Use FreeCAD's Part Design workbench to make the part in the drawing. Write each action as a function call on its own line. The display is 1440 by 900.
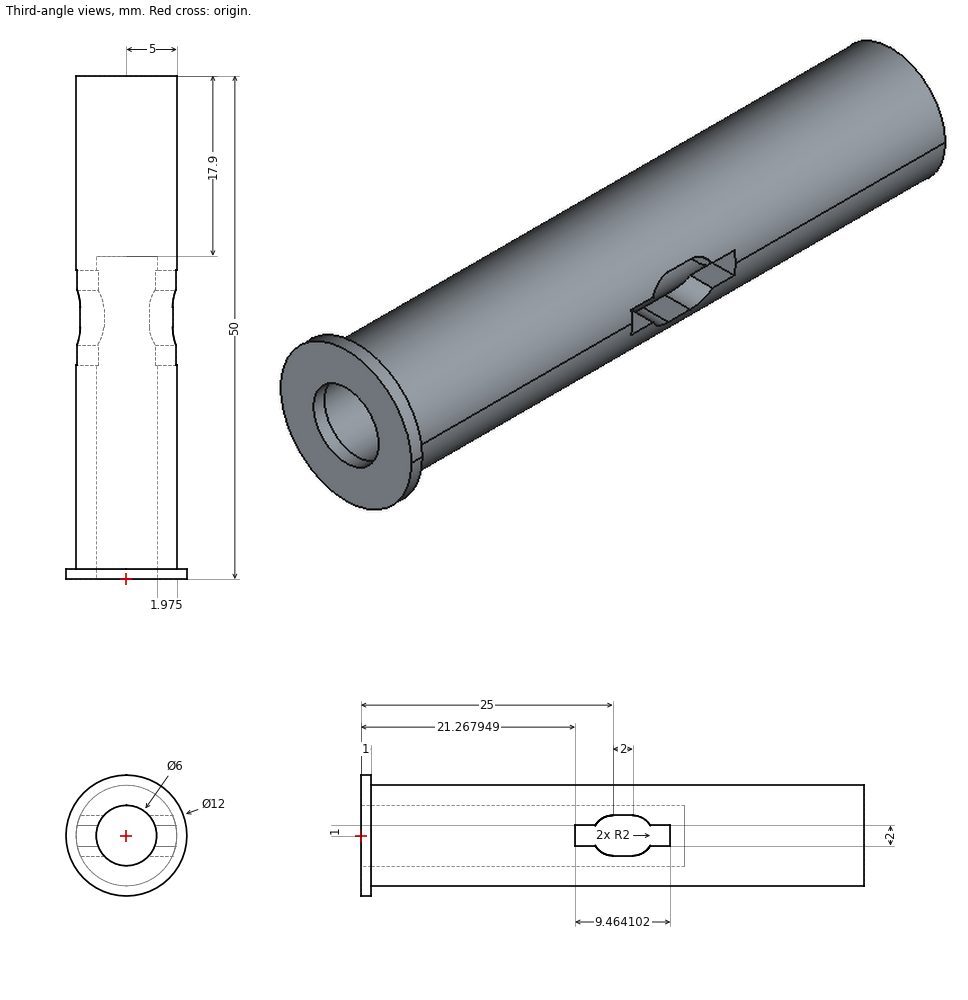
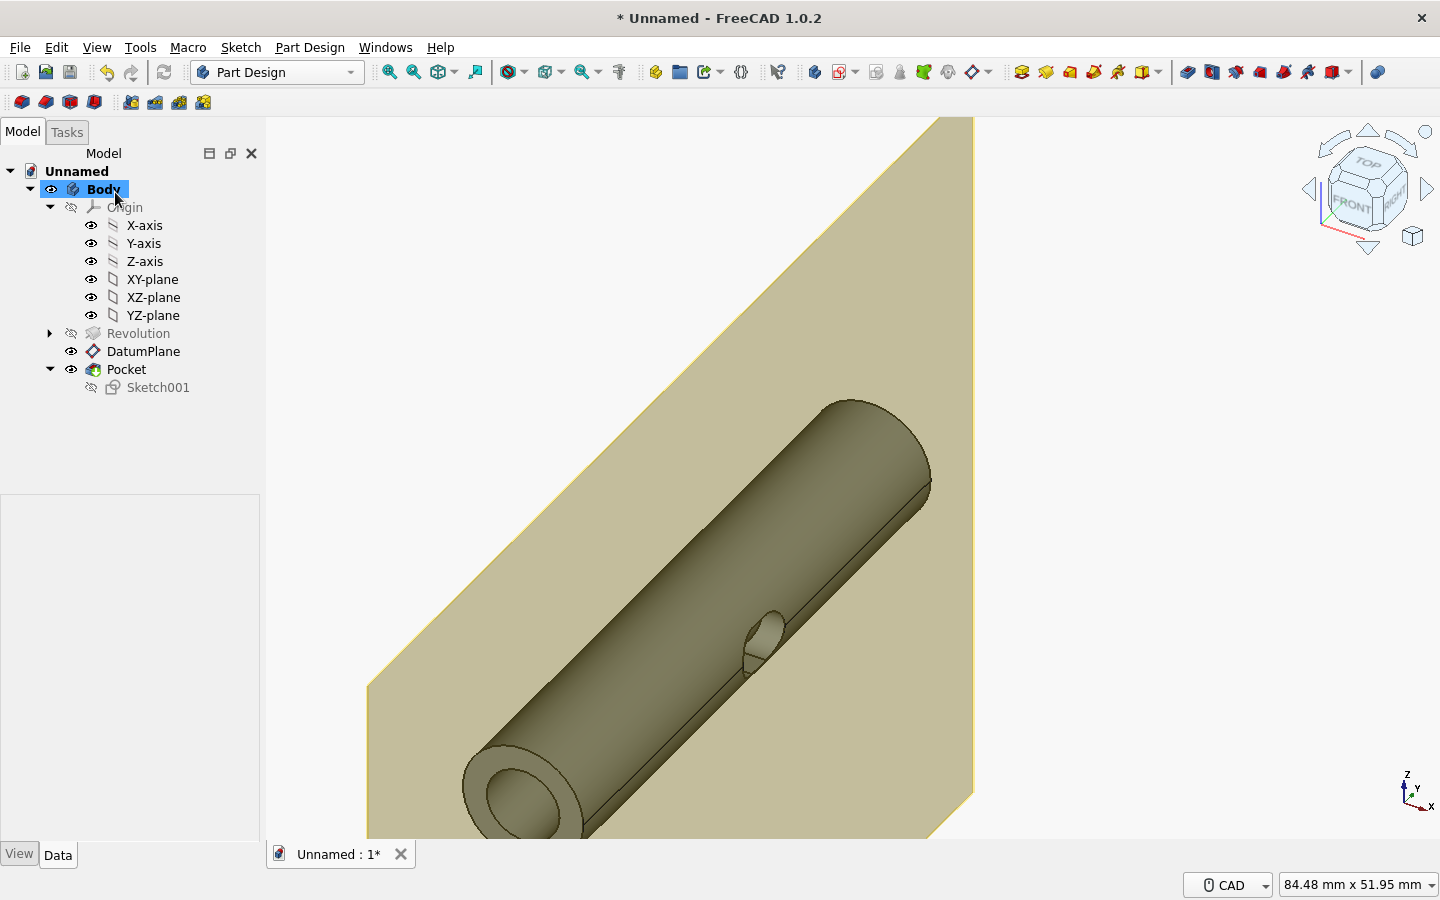
click(116, 351)
key(space)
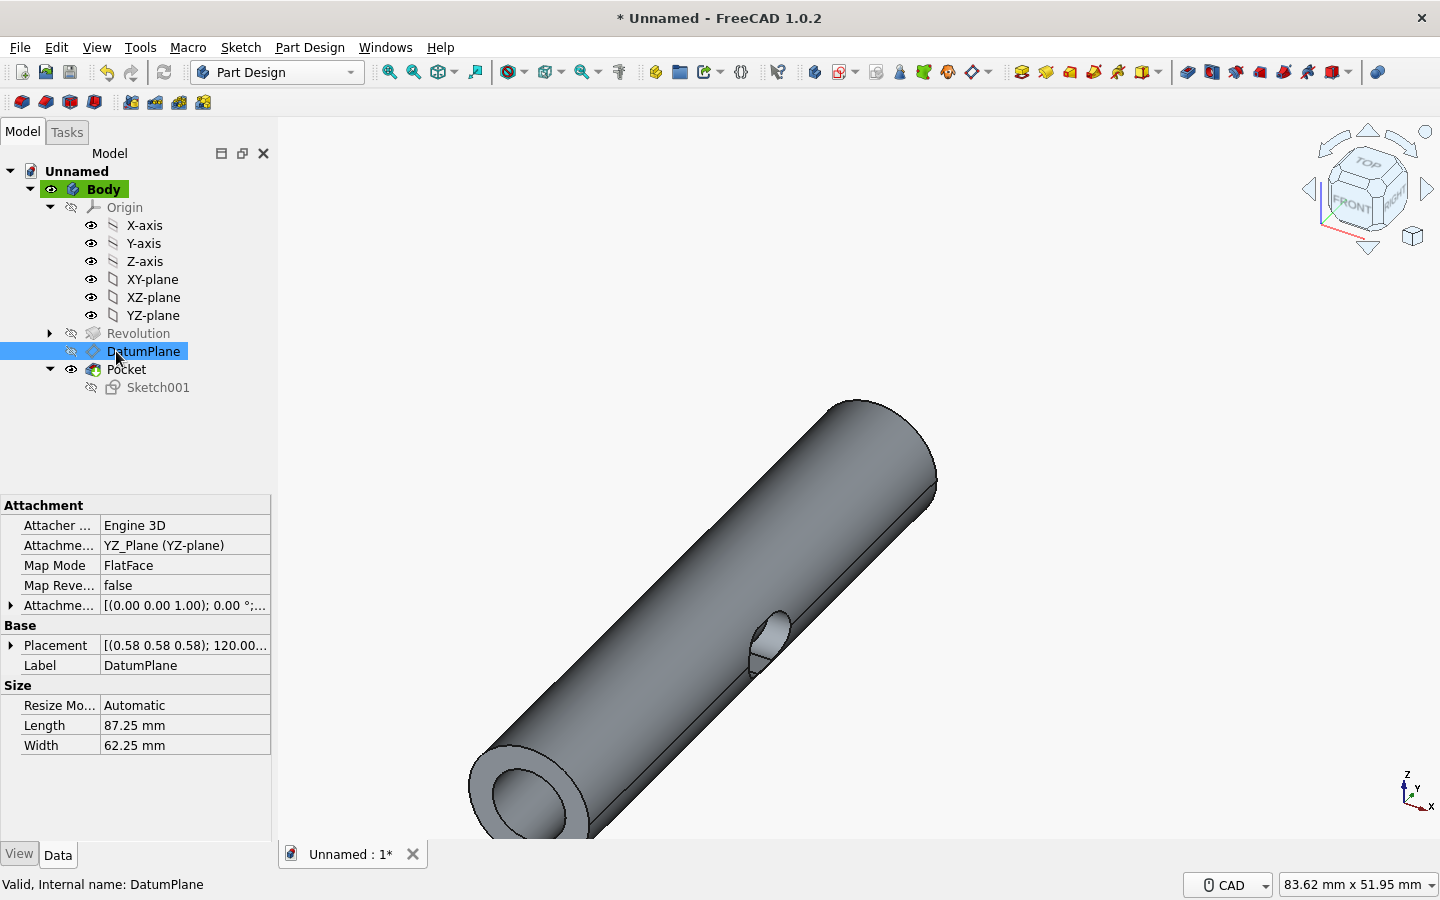
click(390, 72)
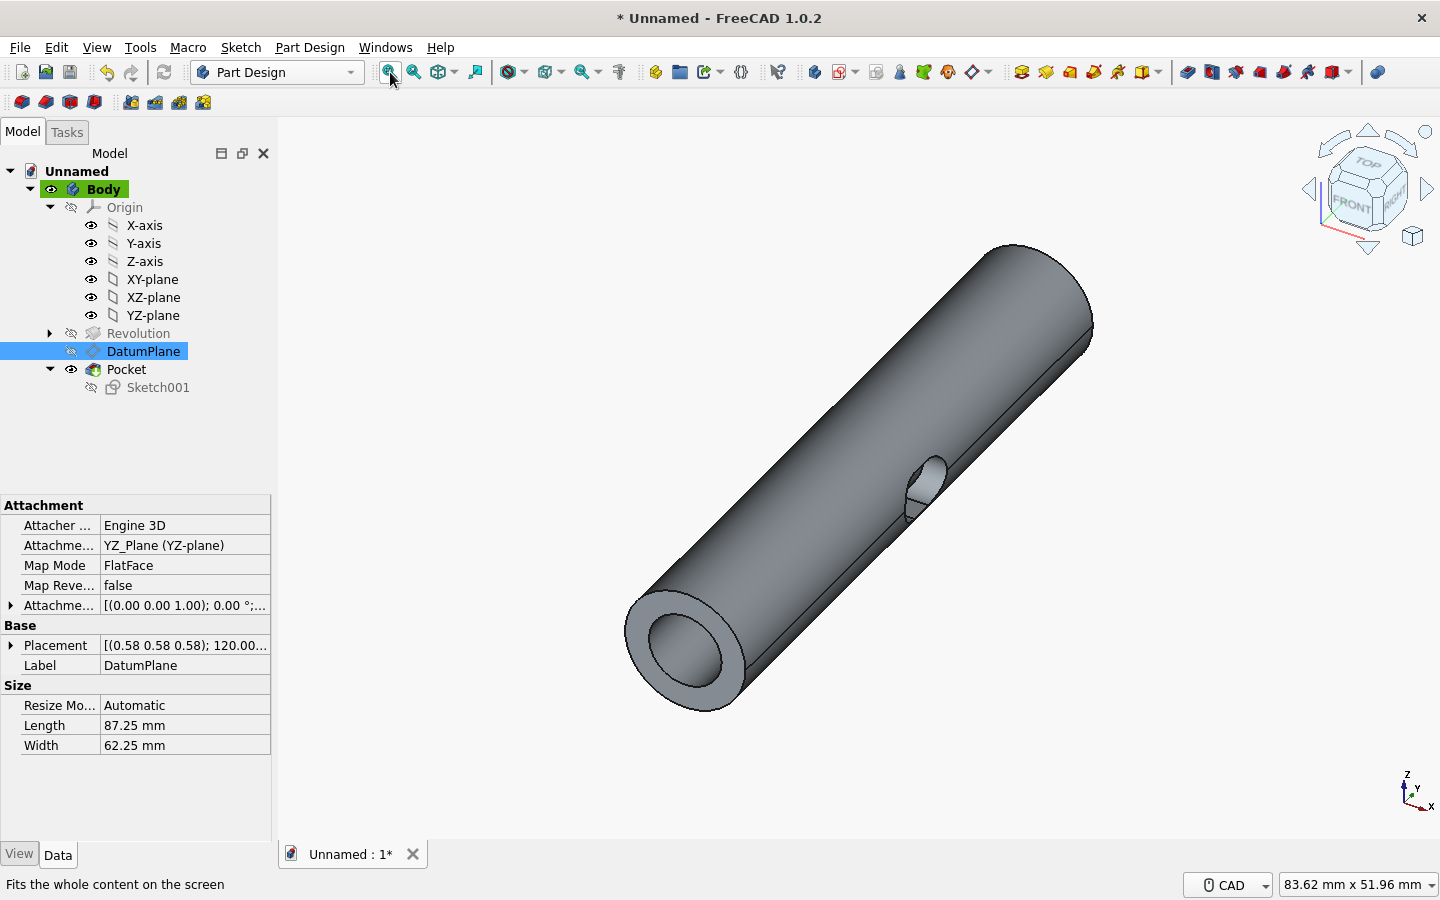
click(318, 799)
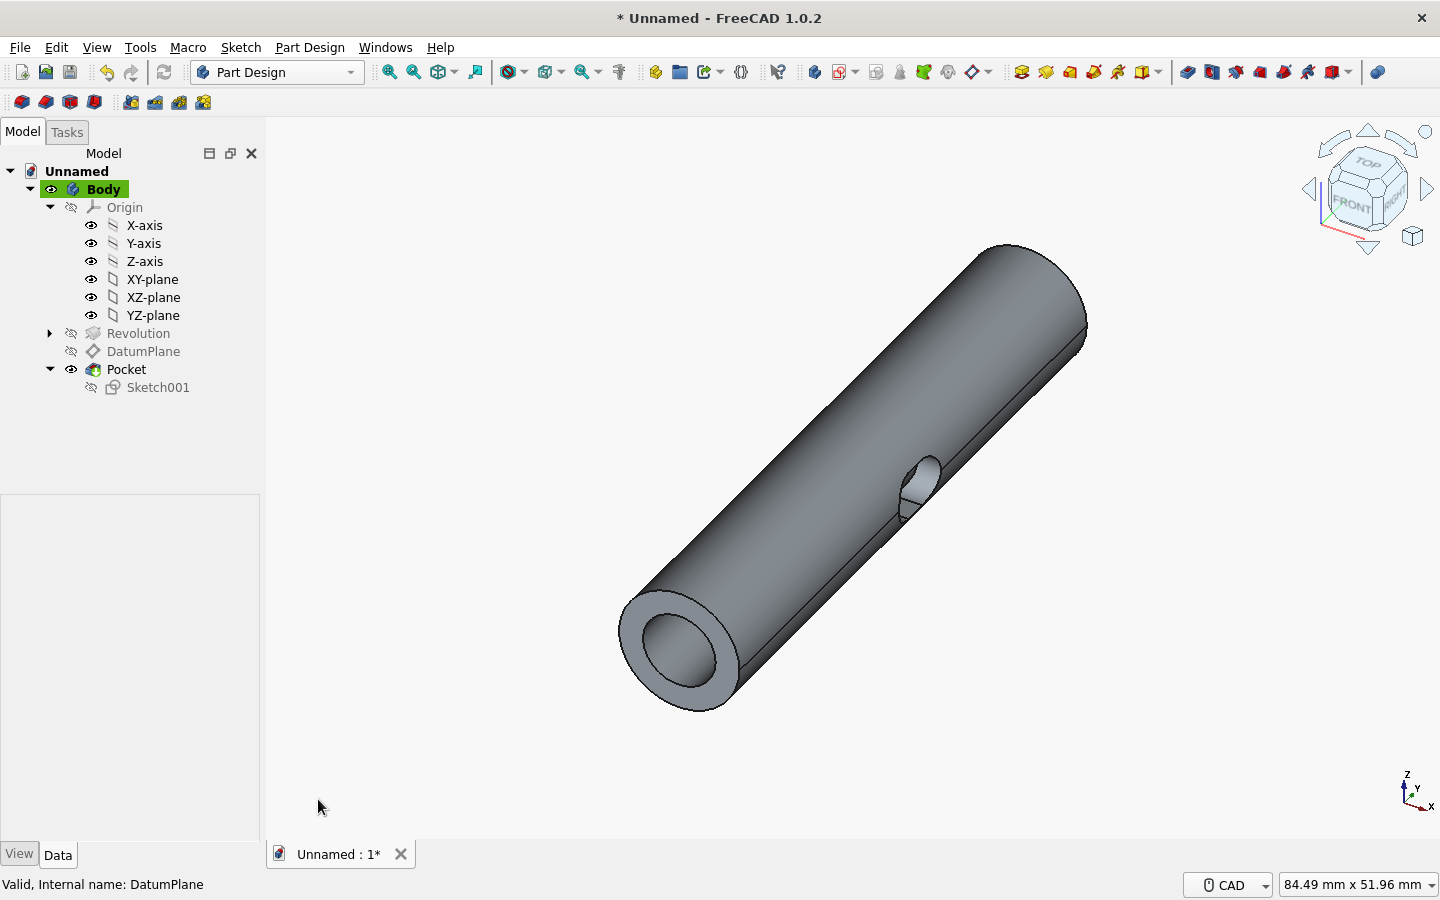
click(840, 72)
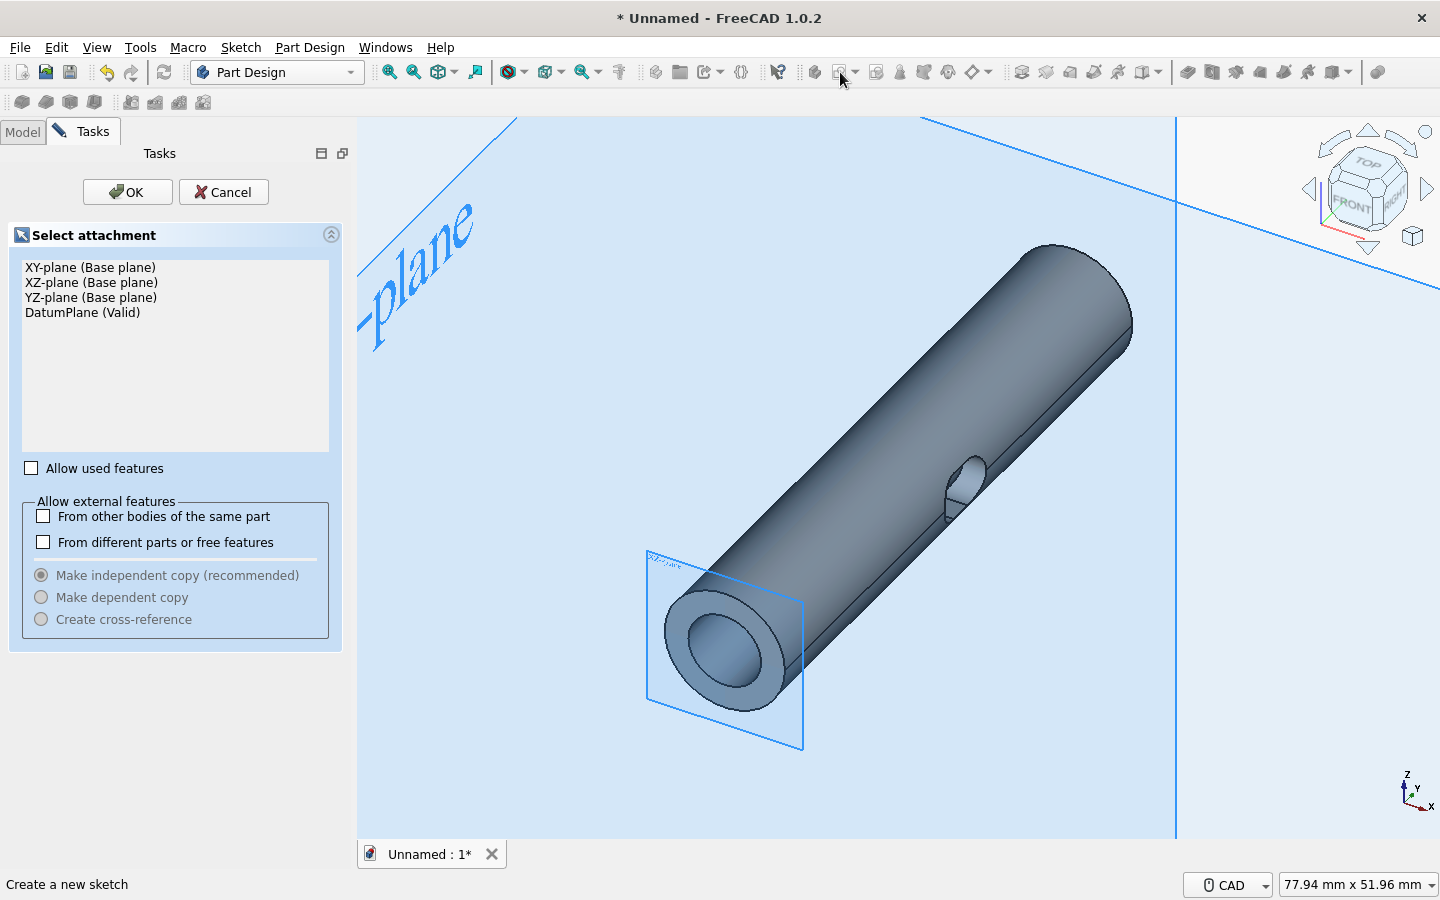
click(82, 282)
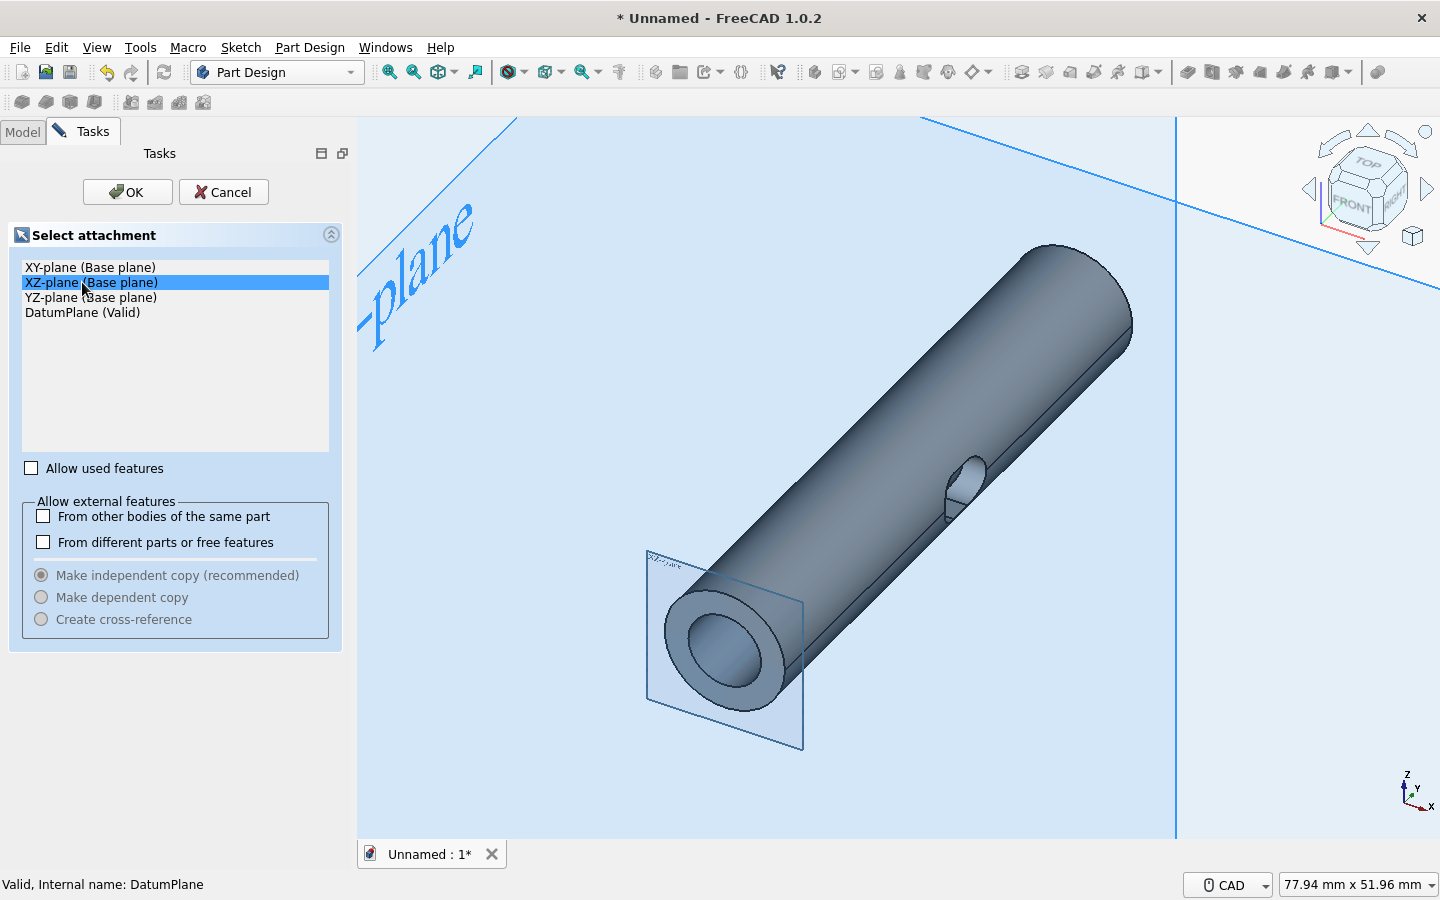
click(128, 192)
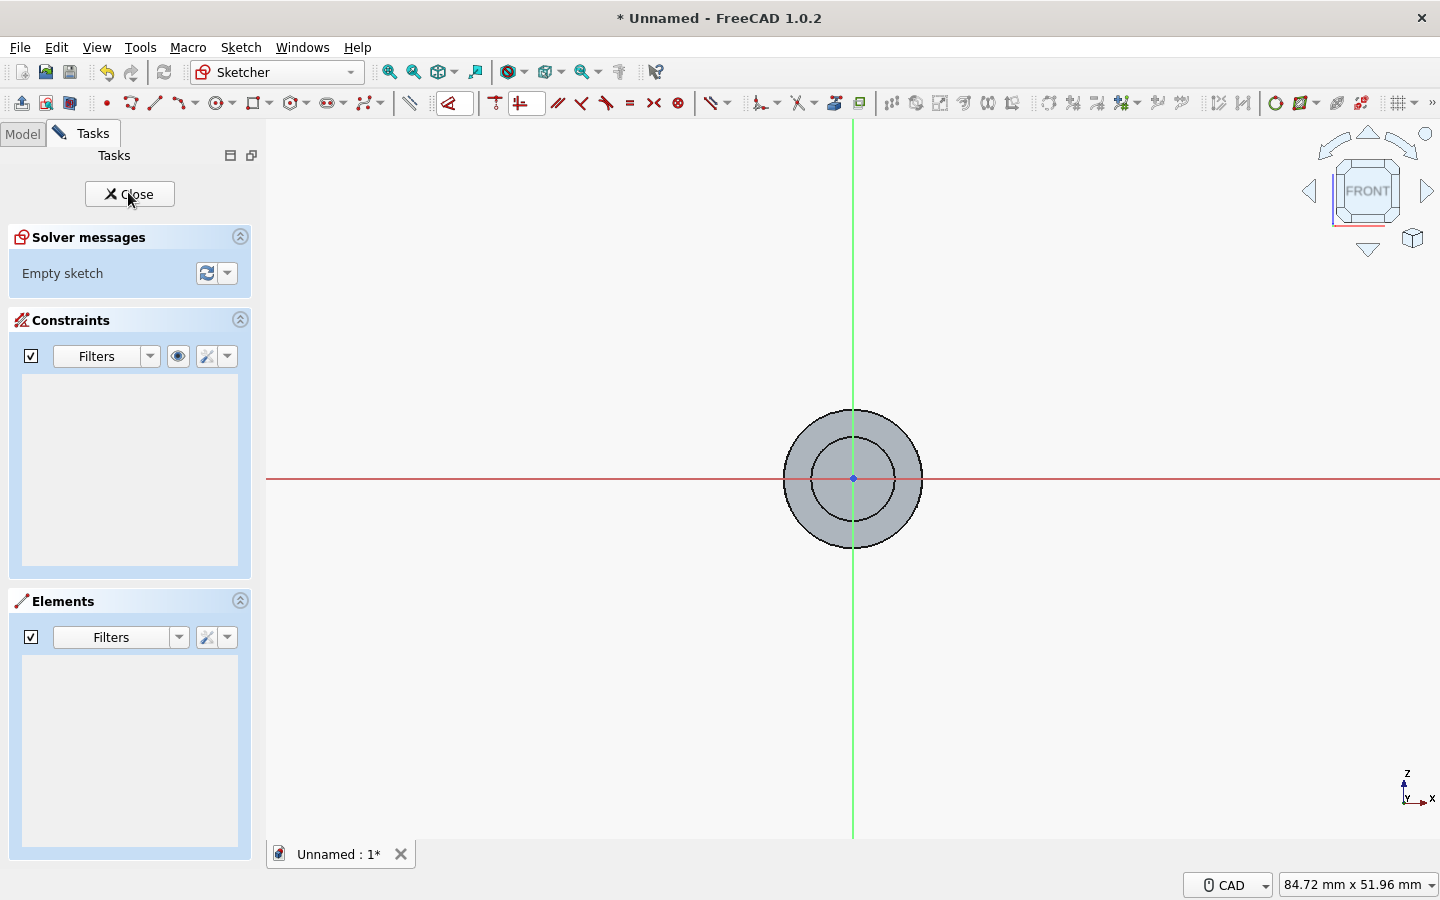
scroll(893, 479, up, 5)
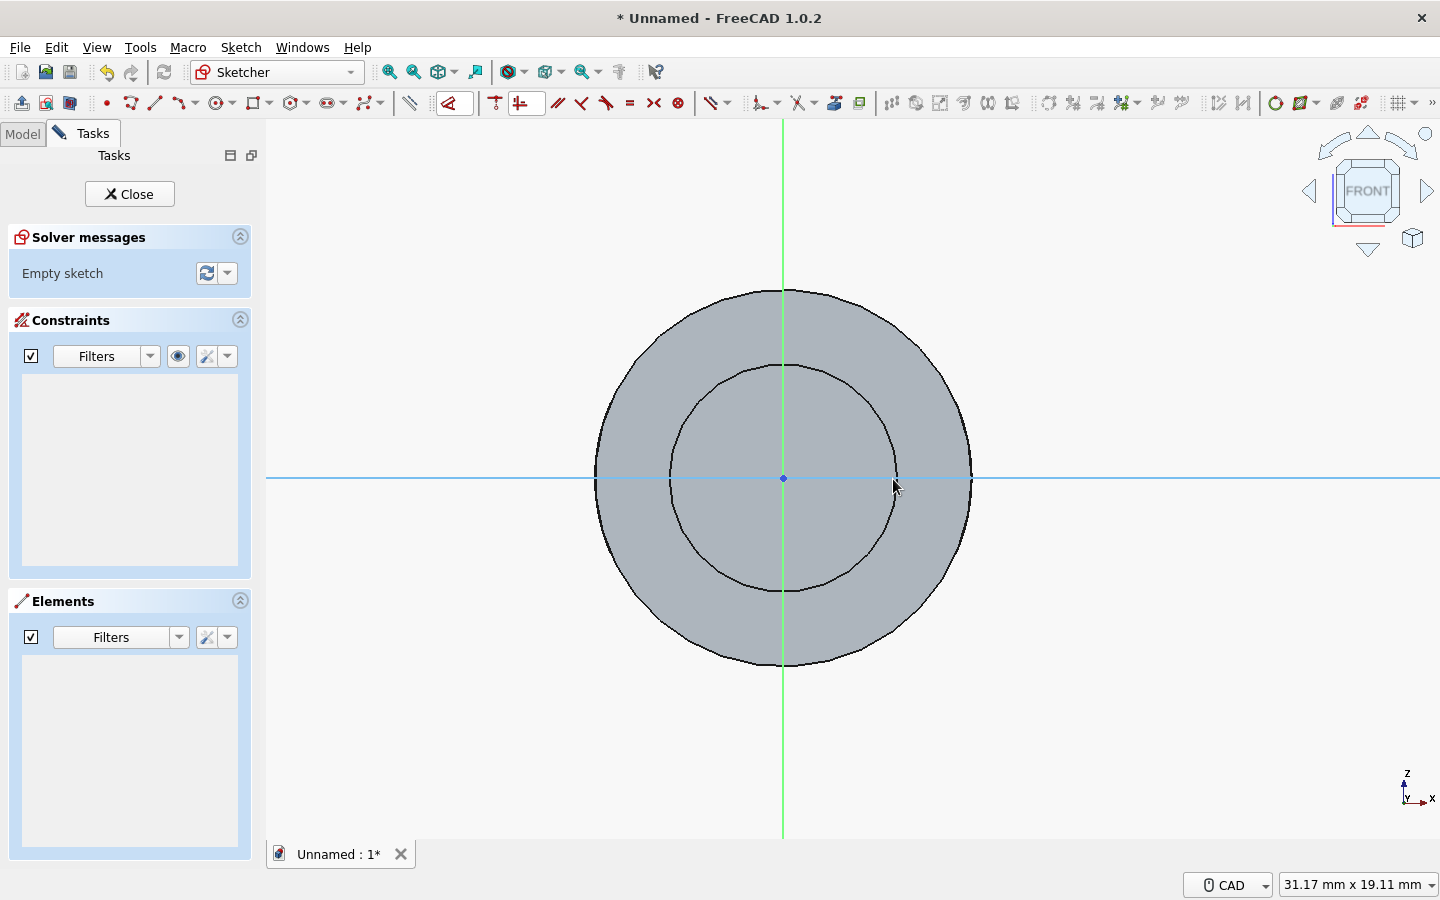
key(g)
key(c)